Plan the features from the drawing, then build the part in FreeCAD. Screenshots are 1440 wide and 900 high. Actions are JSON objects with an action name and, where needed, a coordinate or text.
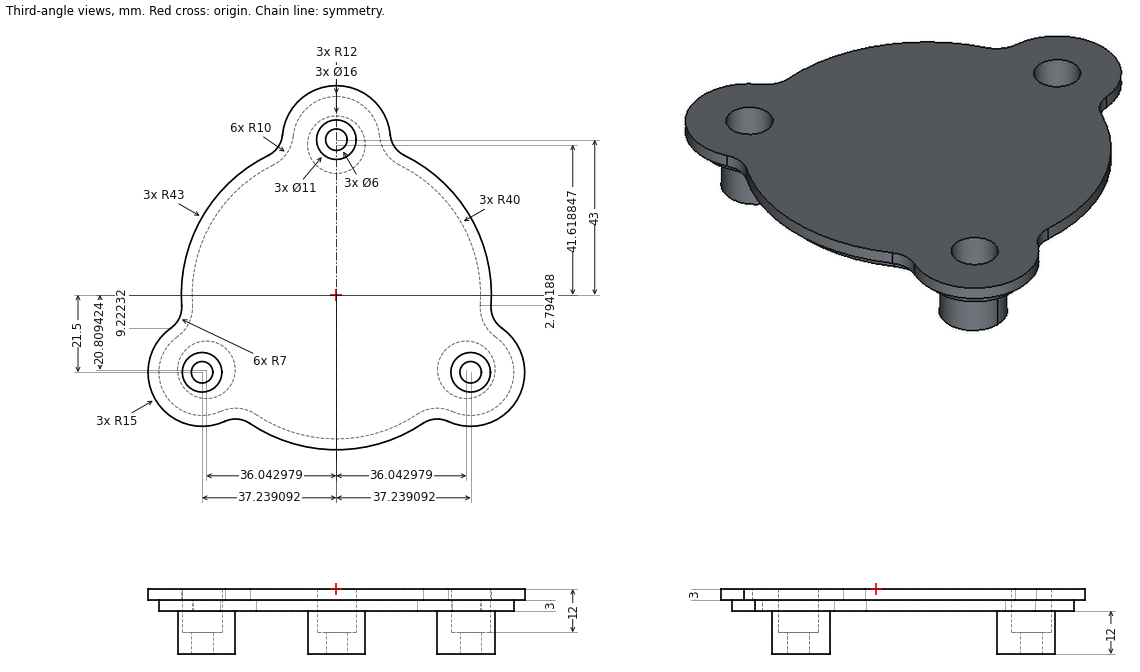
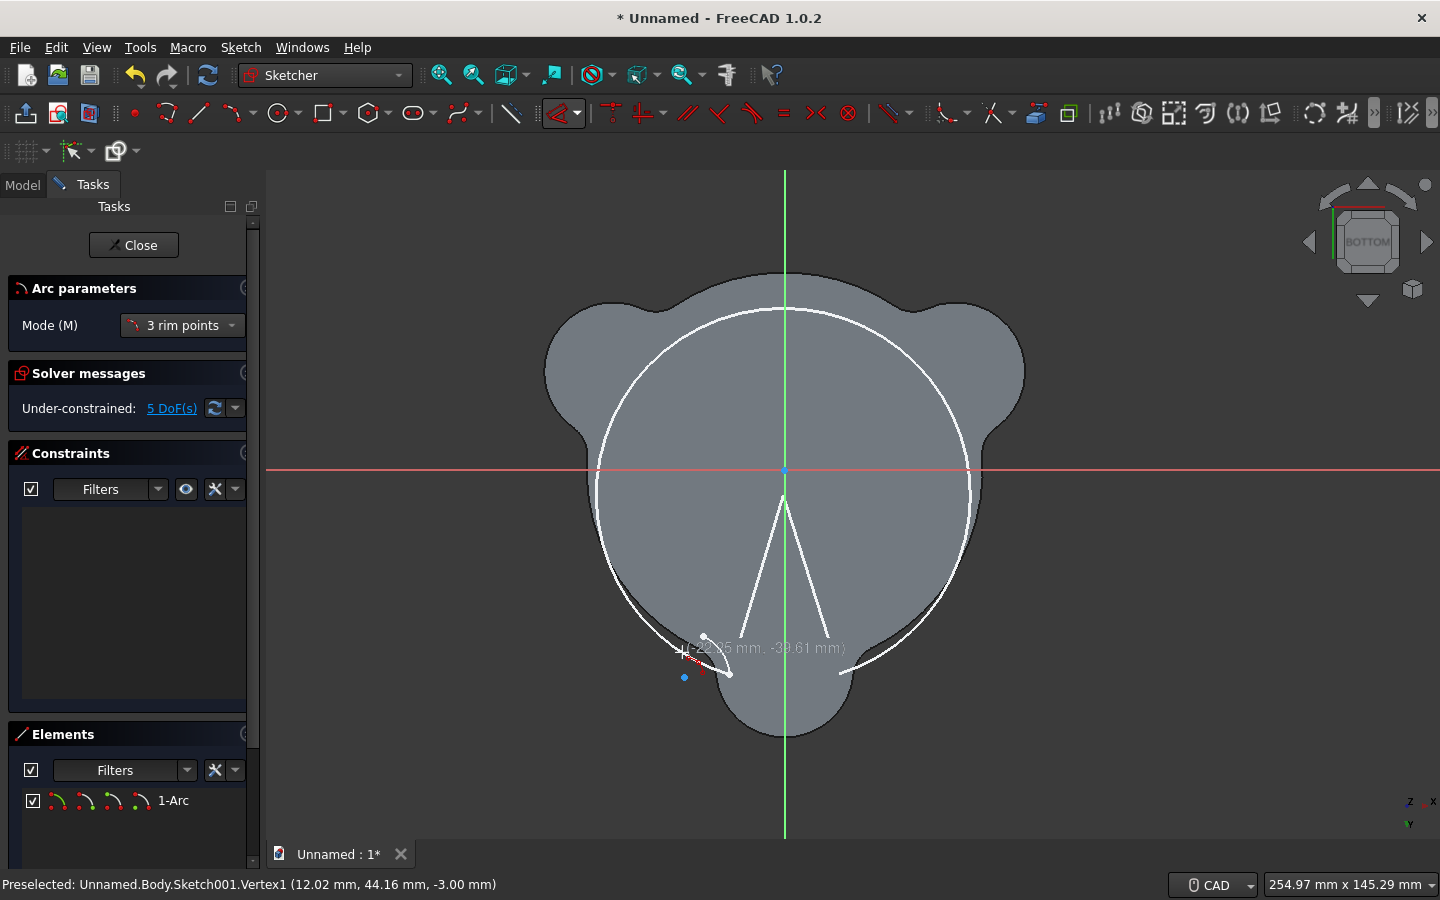
{"action": "left_click", "coordinate": [769, 721]}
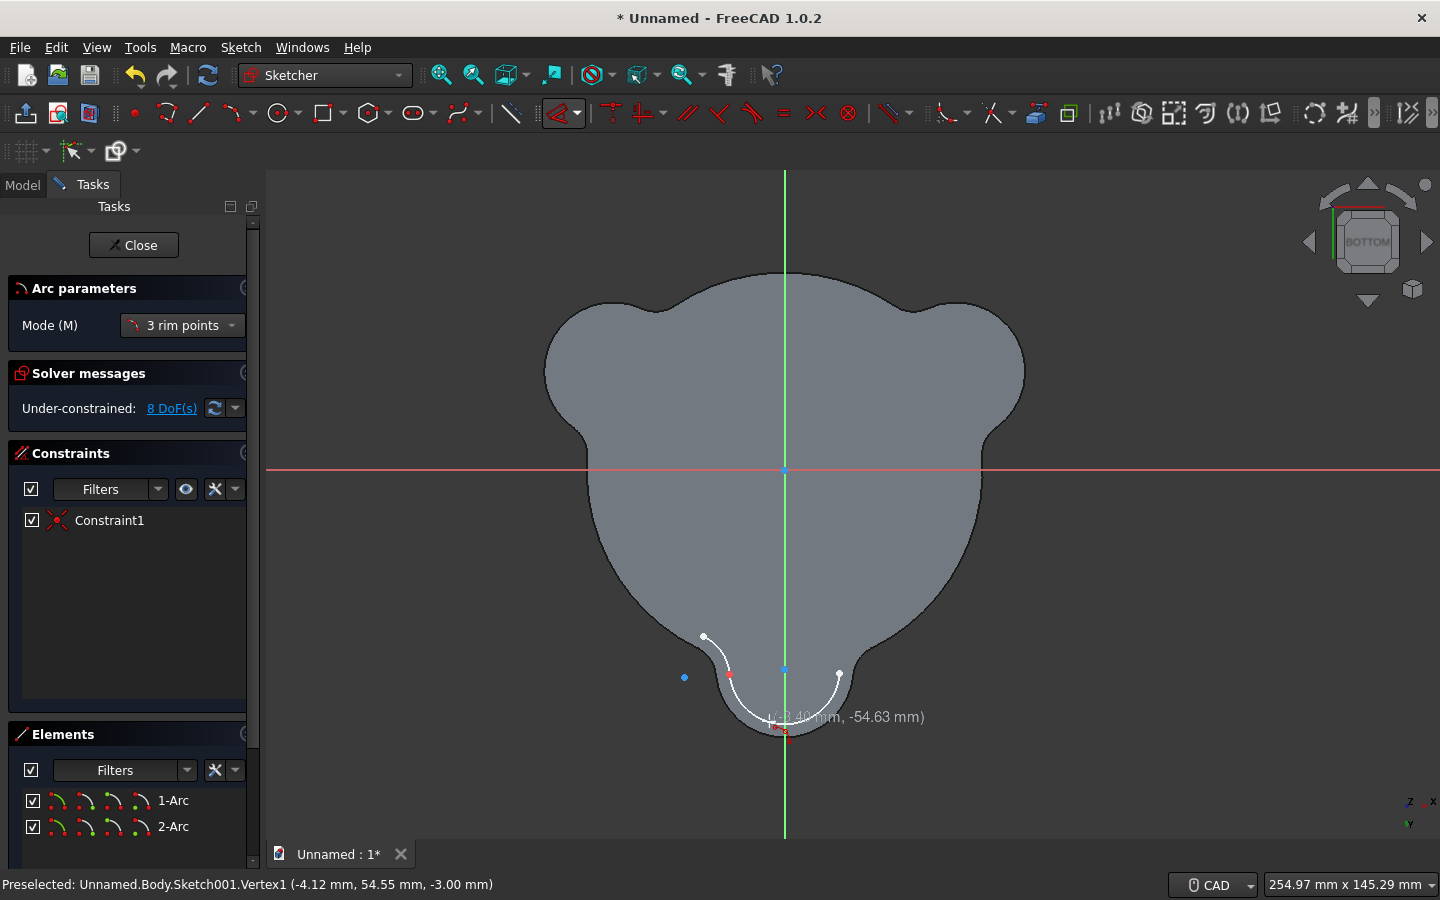
{"action": "left_click", "coordinate": [840, 674]}
{"action": "left_click", "coordinate": [865, 636]}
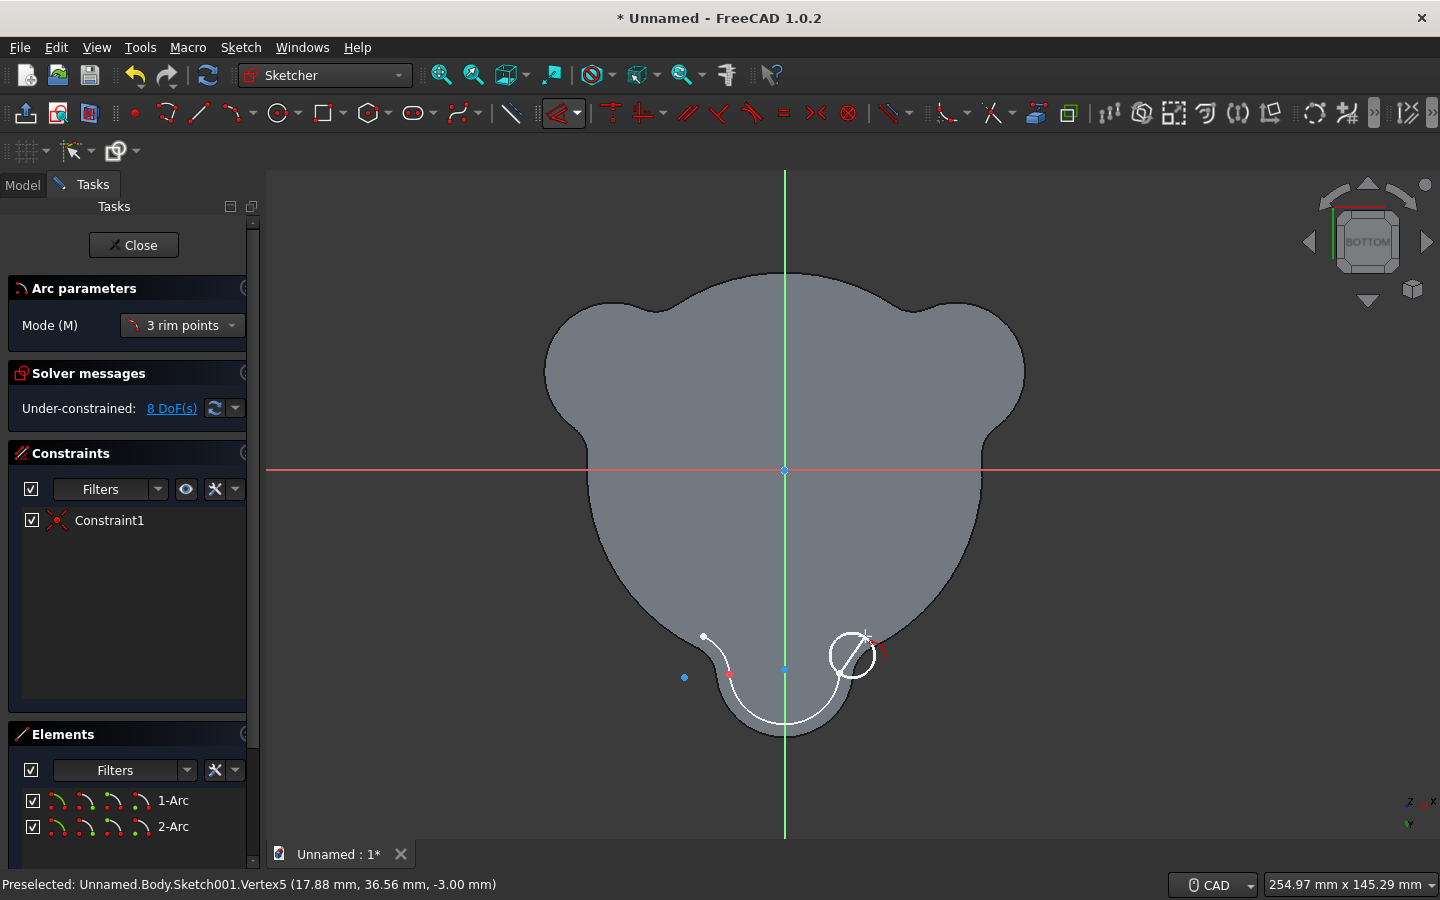
{"action": "scroll", "coordinate": [848, 651], "scroll_direction": "up", "scroll_amount": 5}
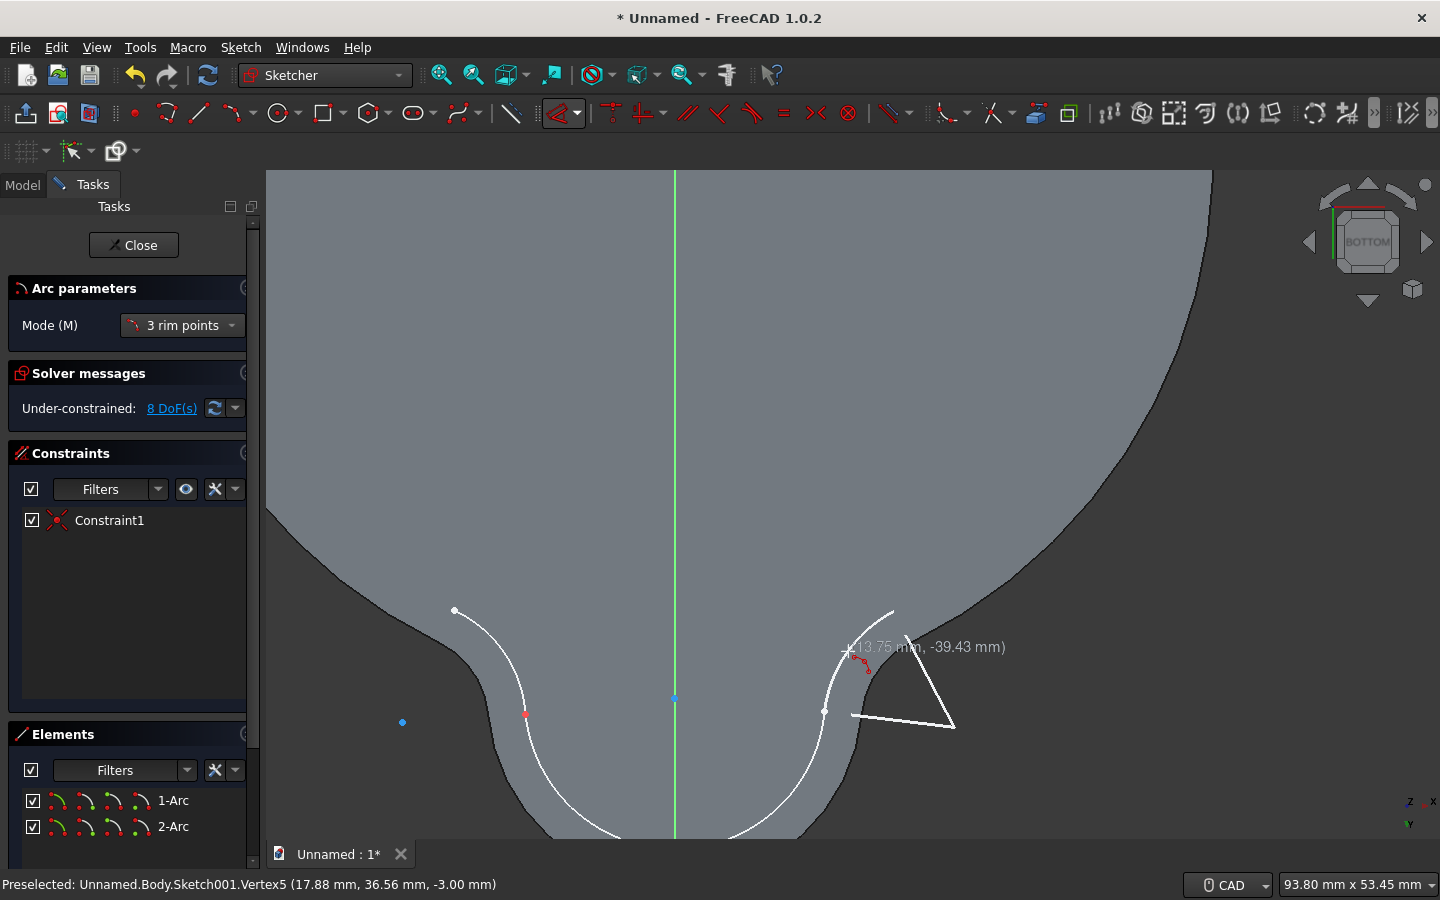
{"action": "left_click", "coordinate": [846, 651]}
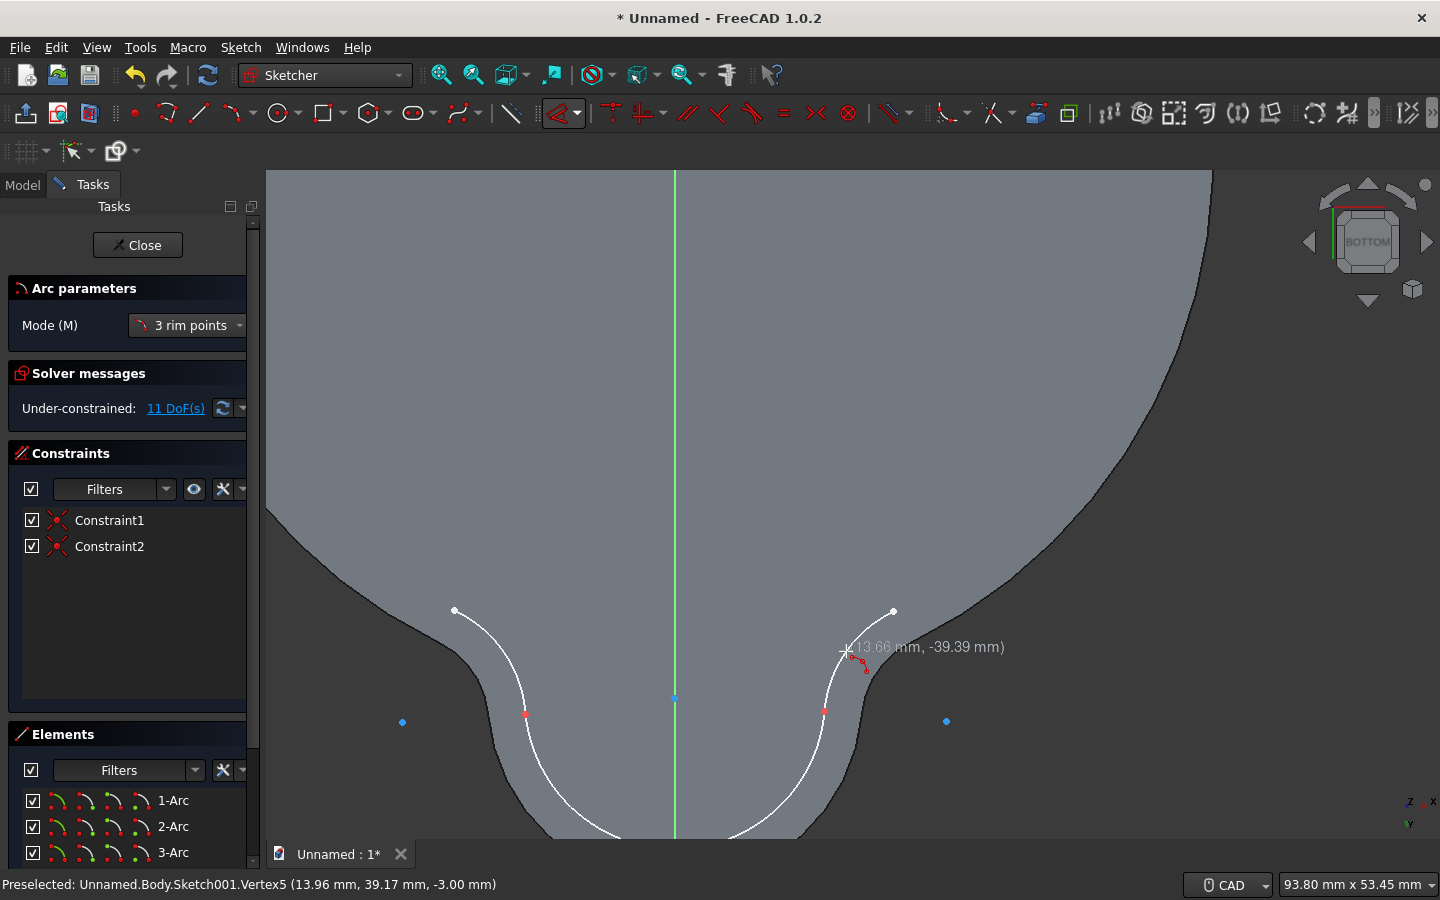
{"action": "left_click", "coordinate": [893, 612]}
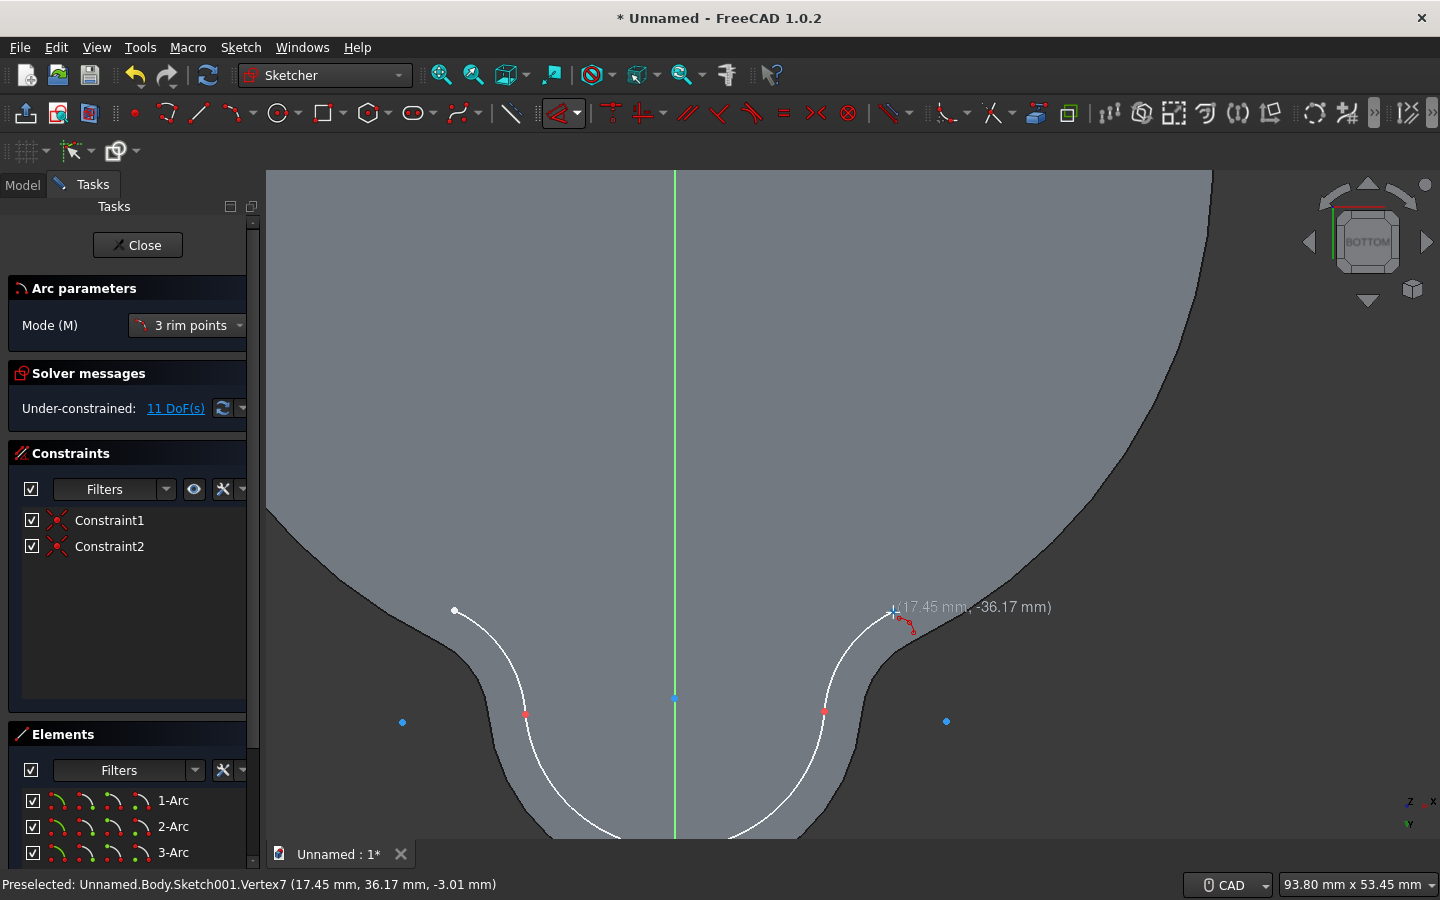
{"action": "scroll", "coordinate": [848, 651], "scroll_direction": "down", "scroll_amount": 5}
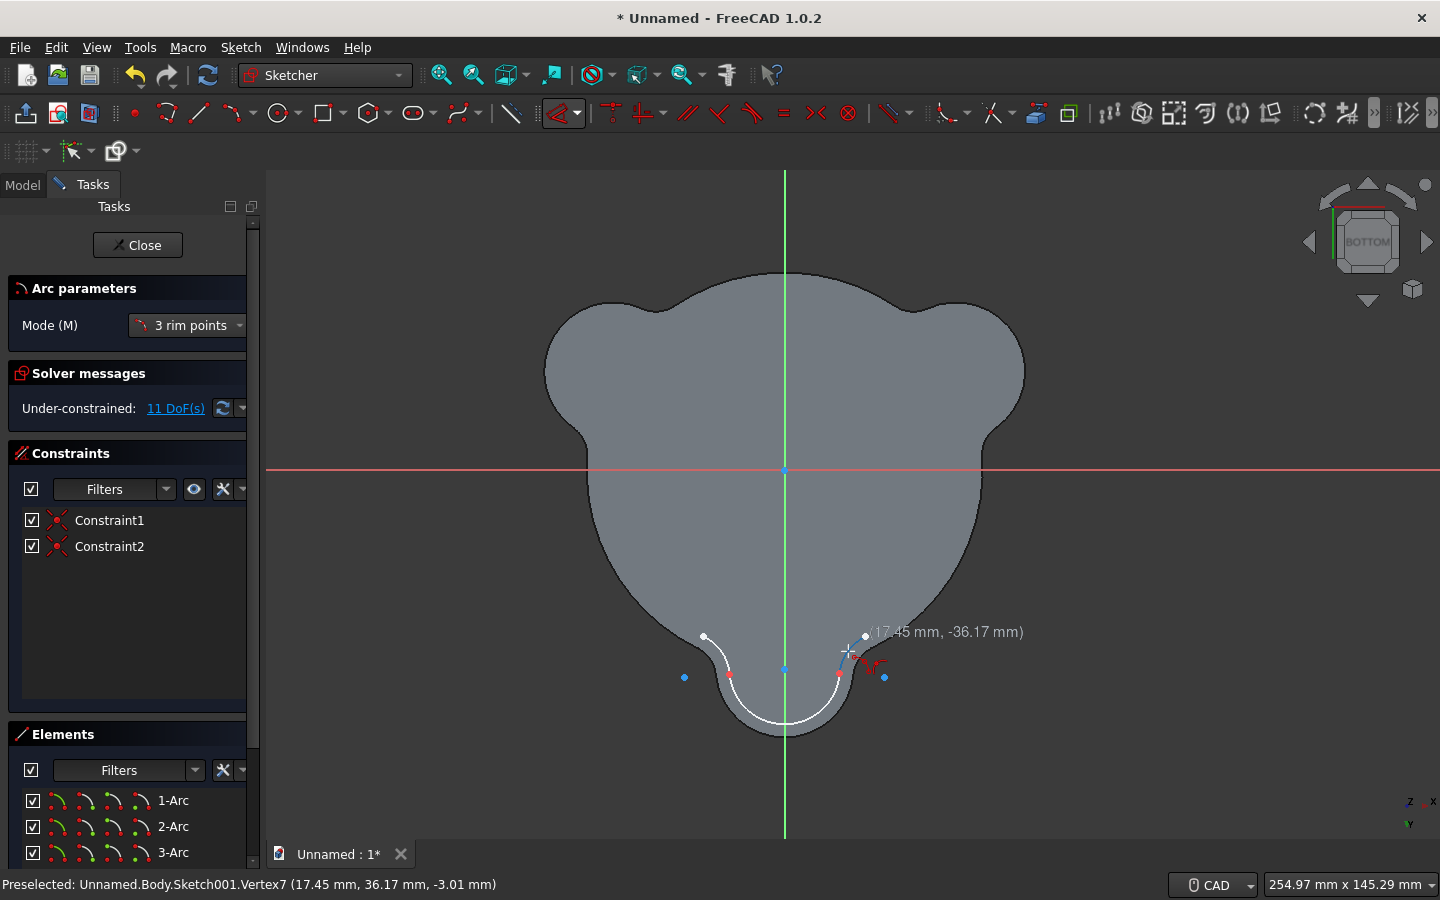
{"action": "scroll", "coordinate": [968, 458], "scroll_direction": "up", "scroll_amount": 2}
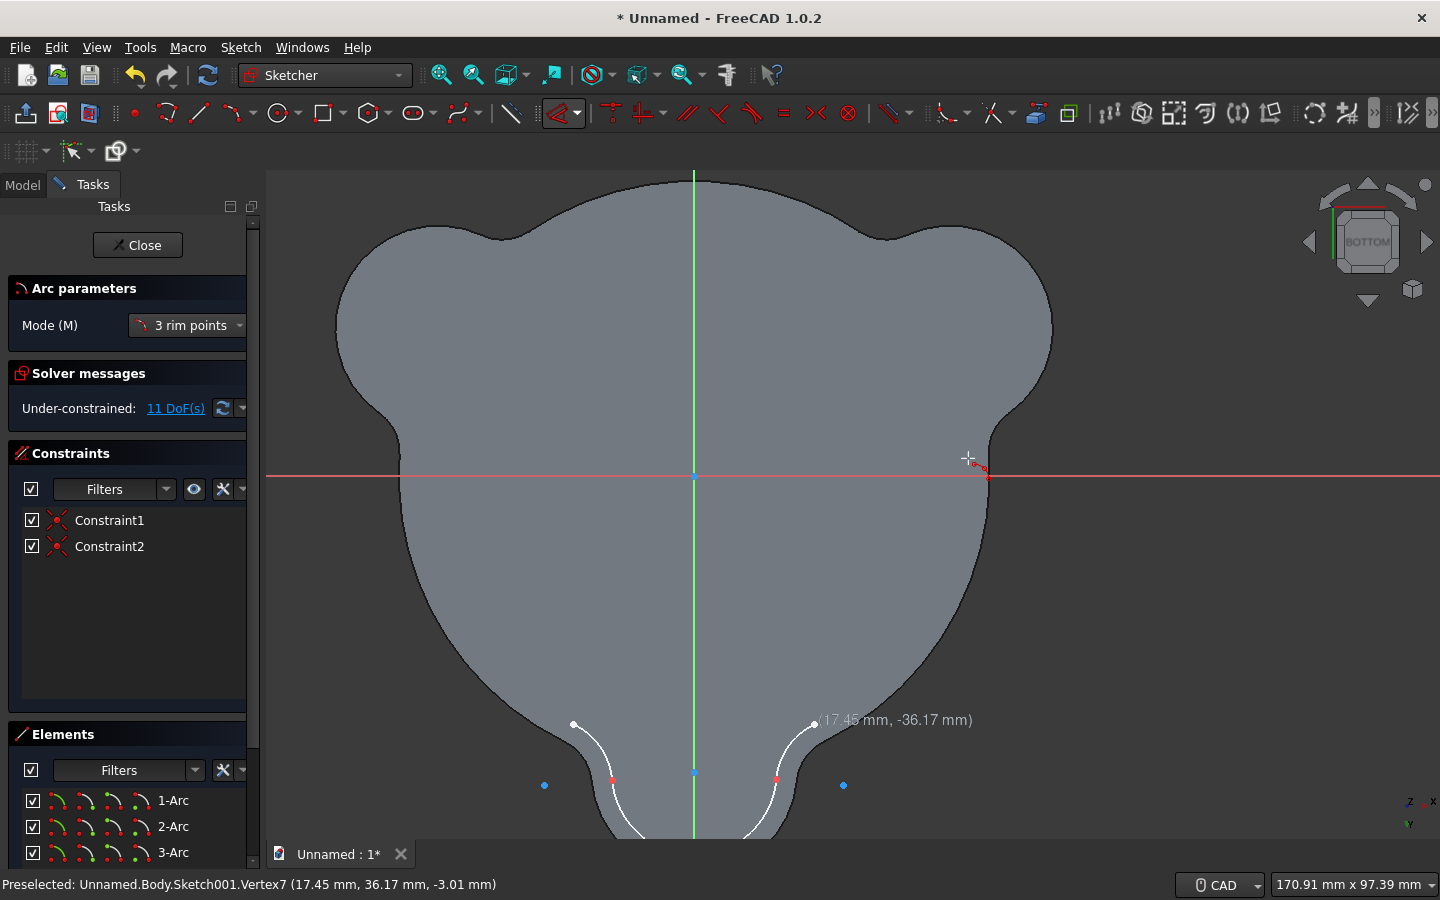
{"action": "left_click", "coordinate": [968, 457]}
{"action": "left_click", "coordinate": [932, 614]}